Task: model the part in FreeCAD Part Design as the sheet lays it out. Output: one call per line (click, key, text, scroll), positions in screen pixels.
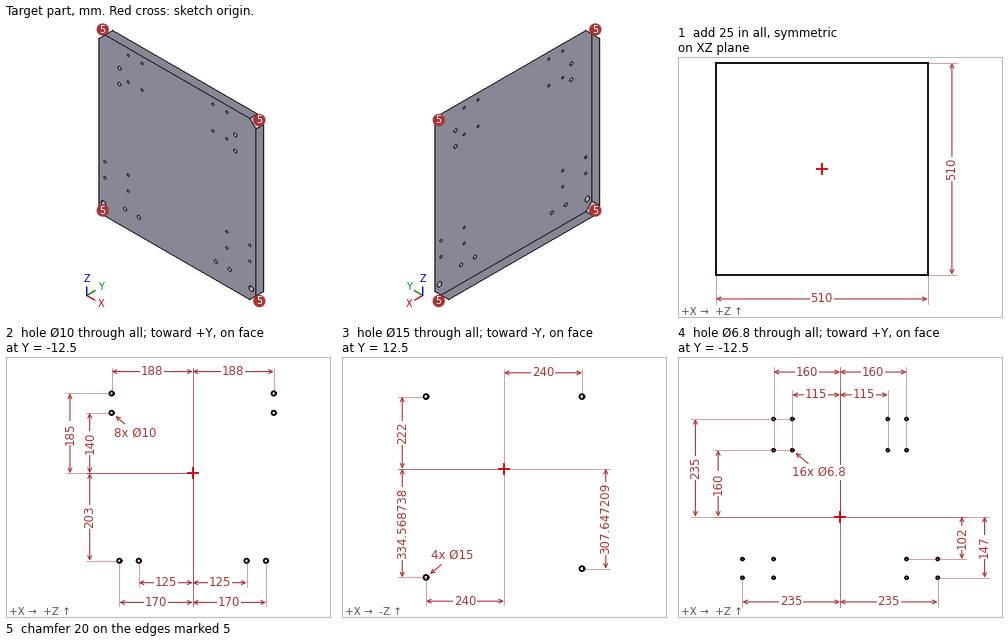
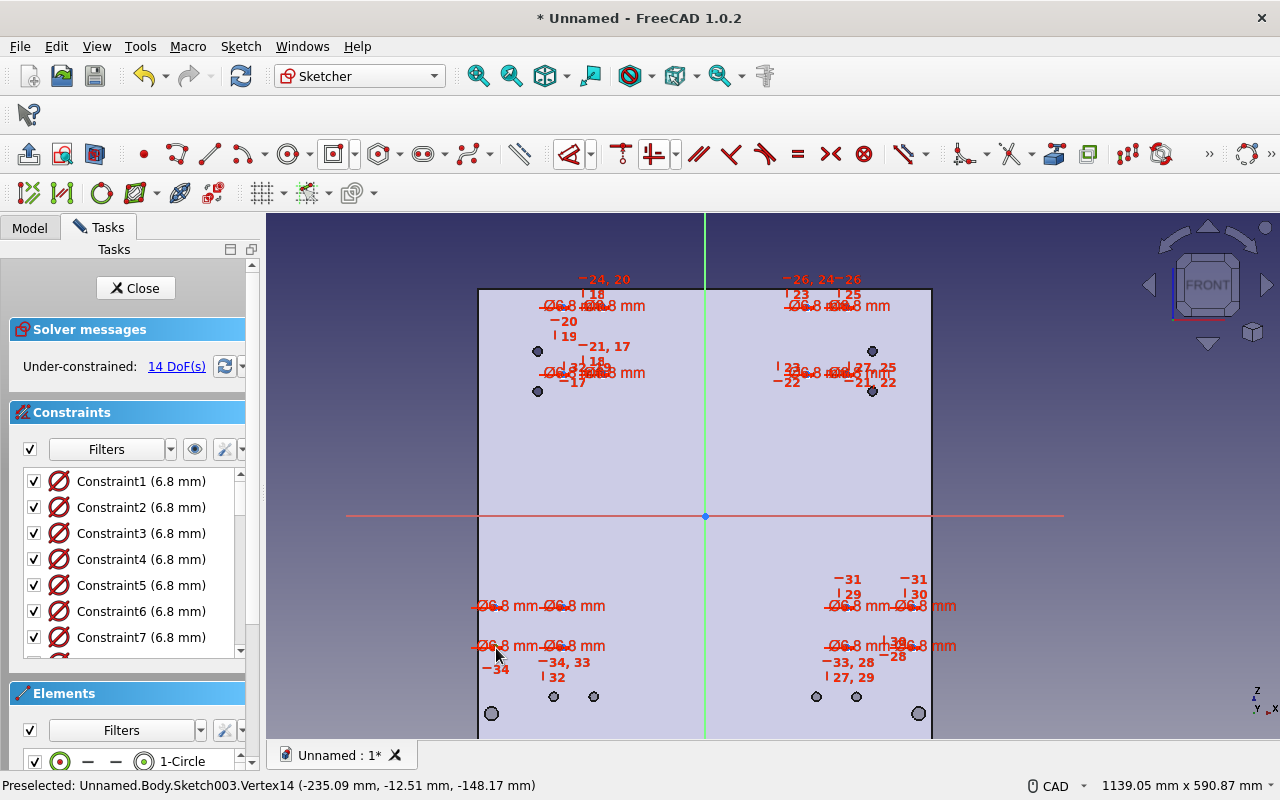
click(496, 608)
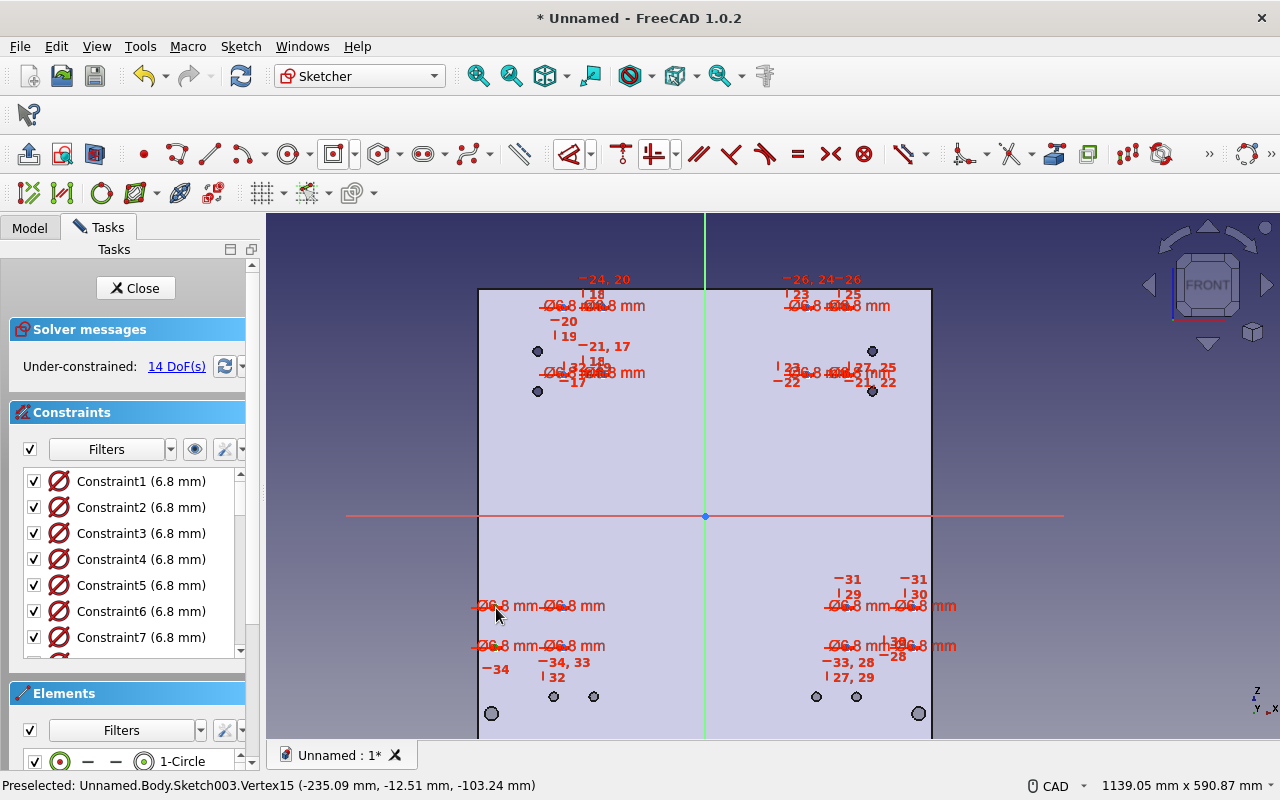
click(676, 154)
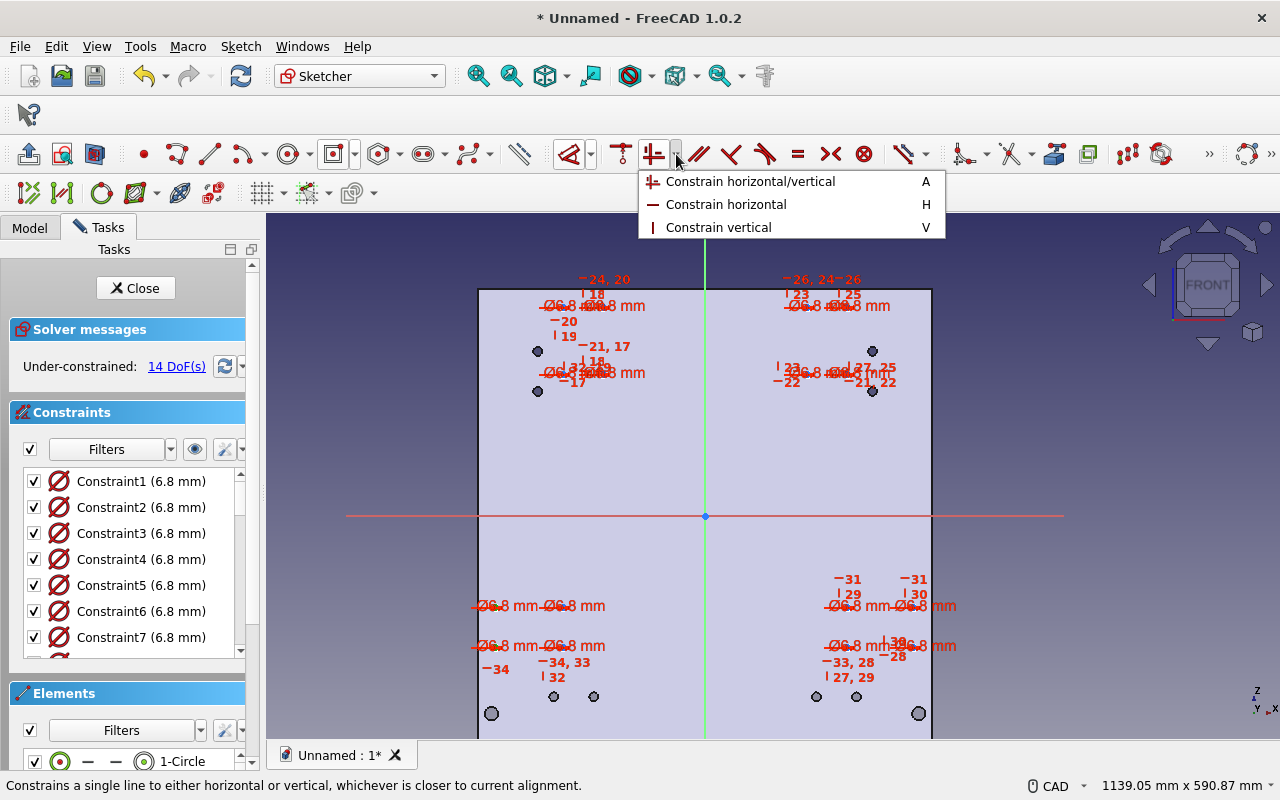
click(792, 228)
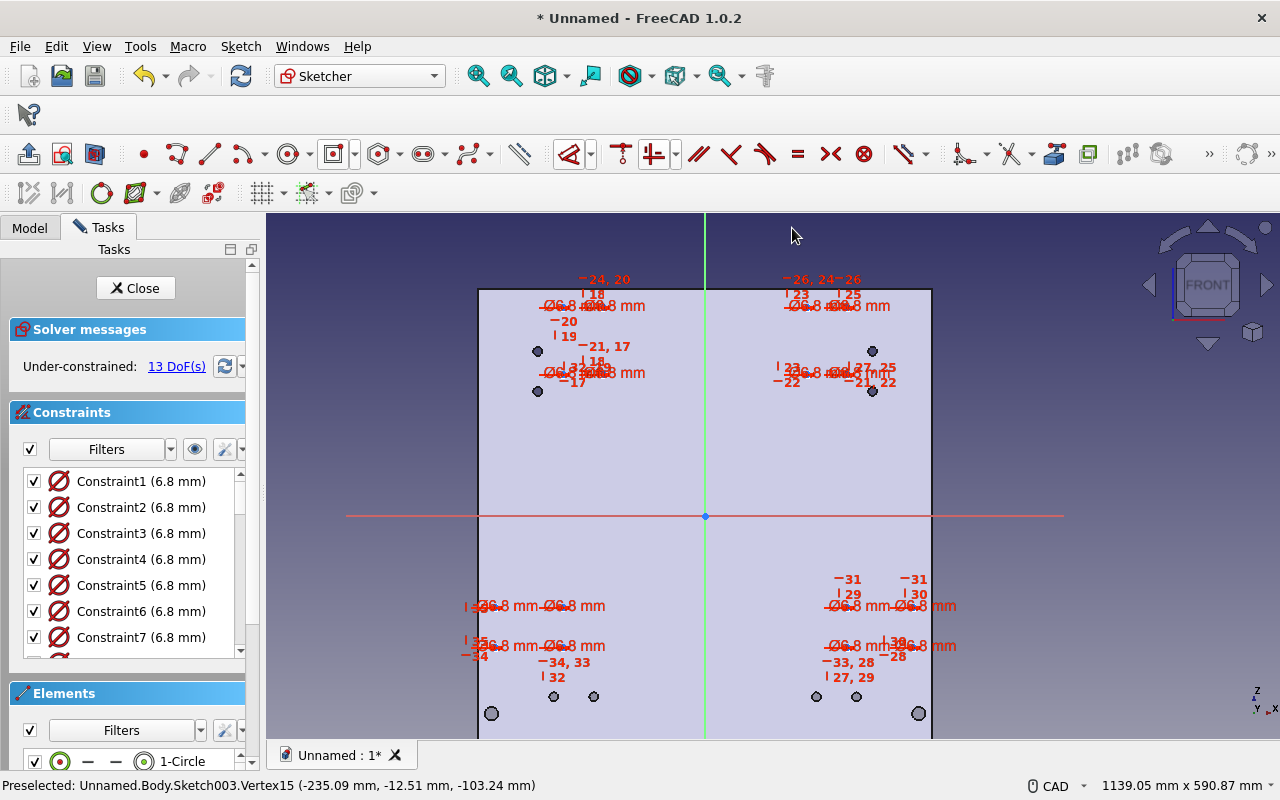
click(563, 648)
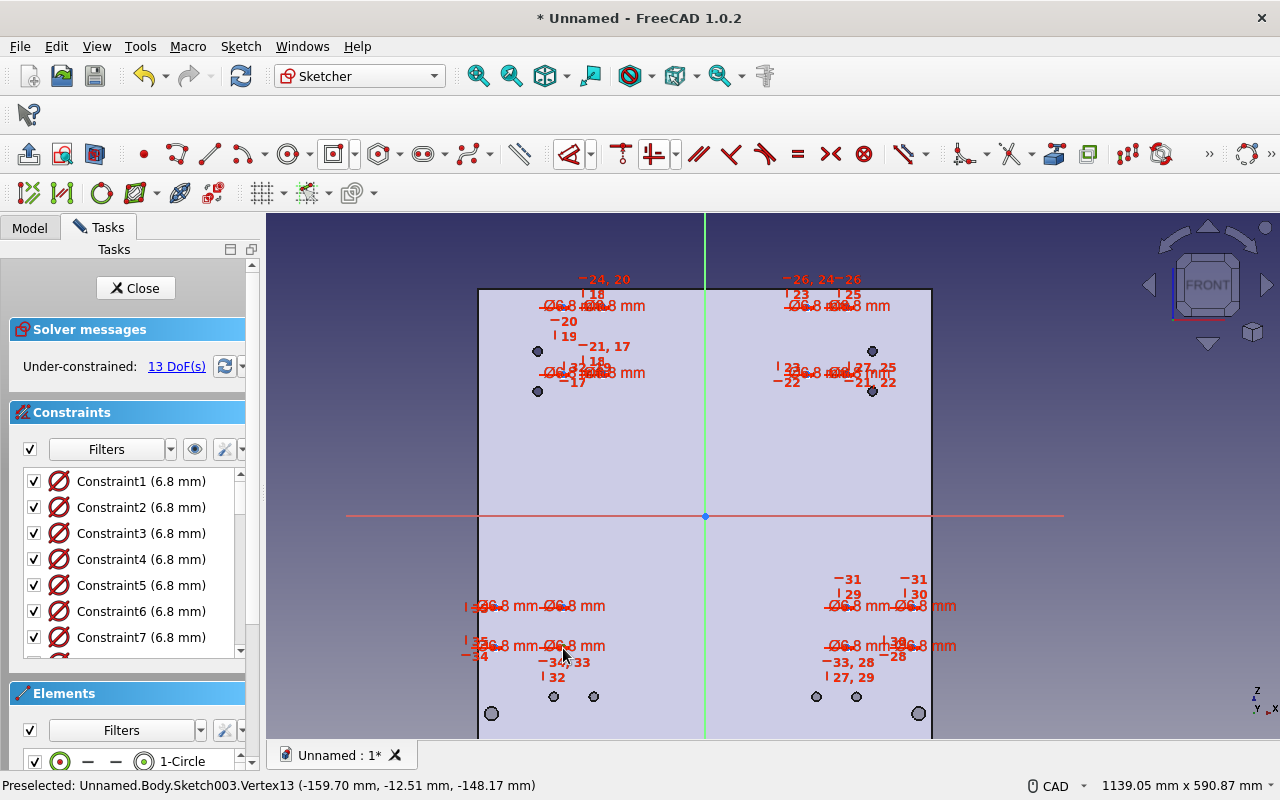
click(563, 608)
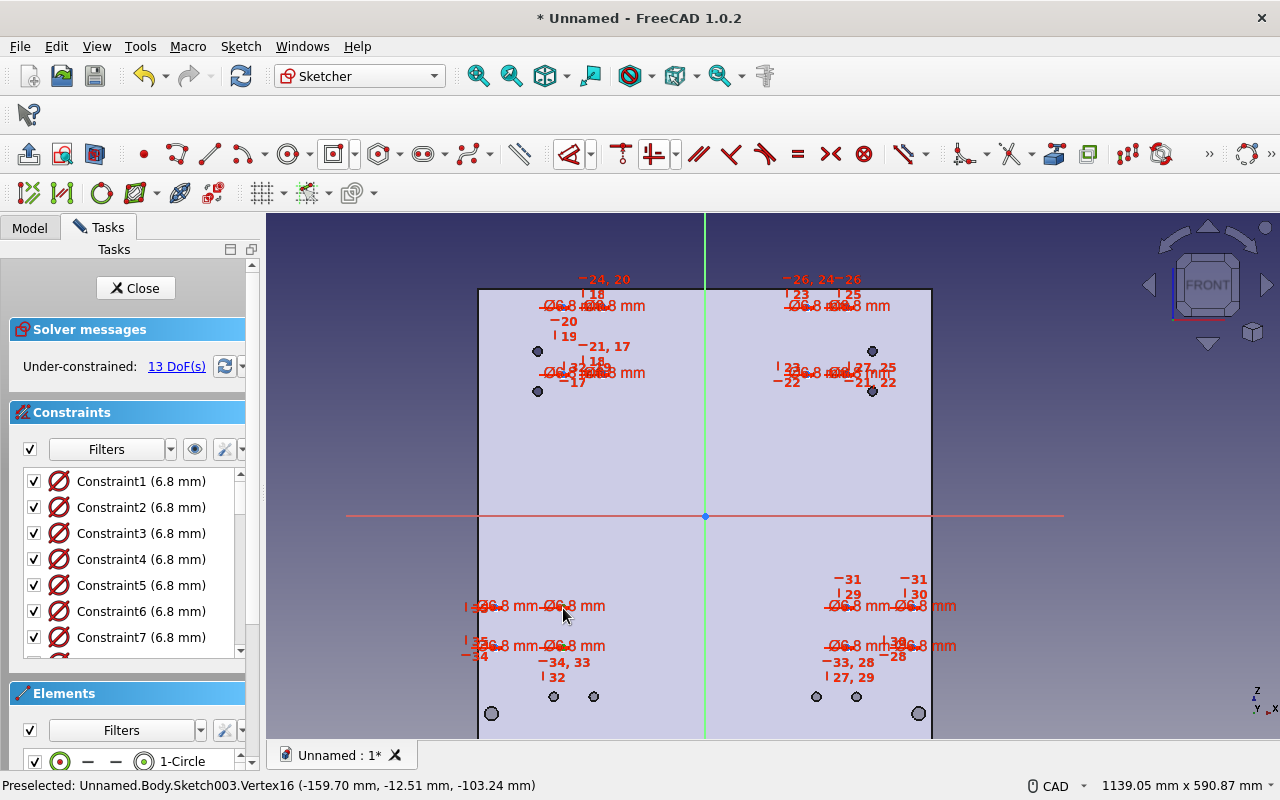
key(v)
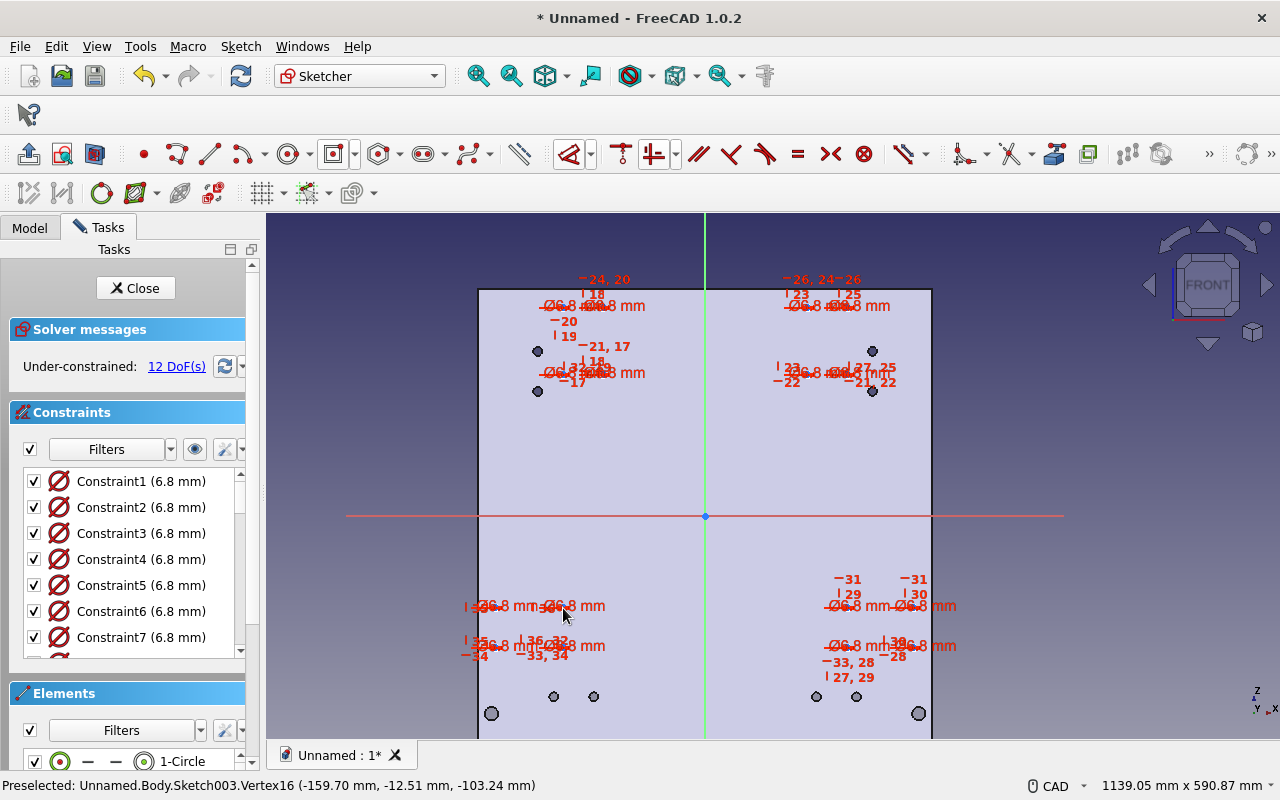
click(496, 608)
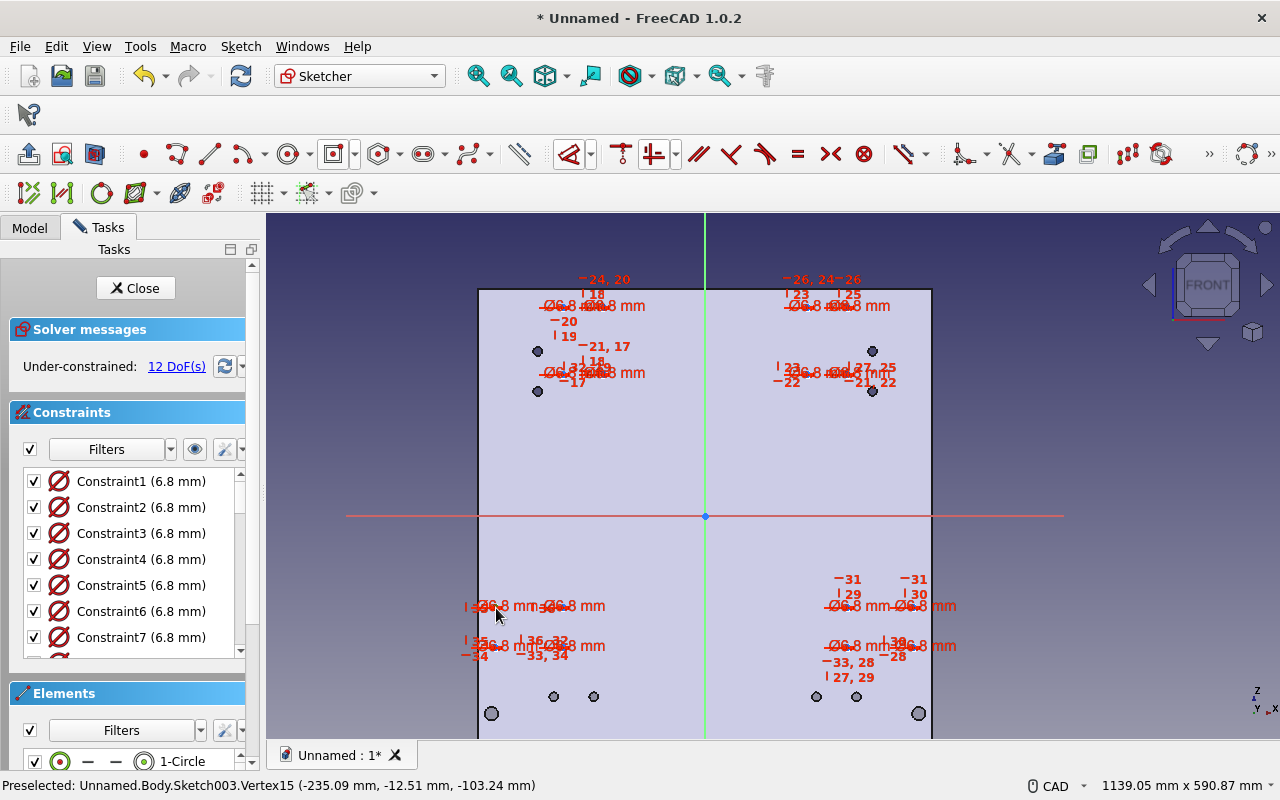
click(563, 608)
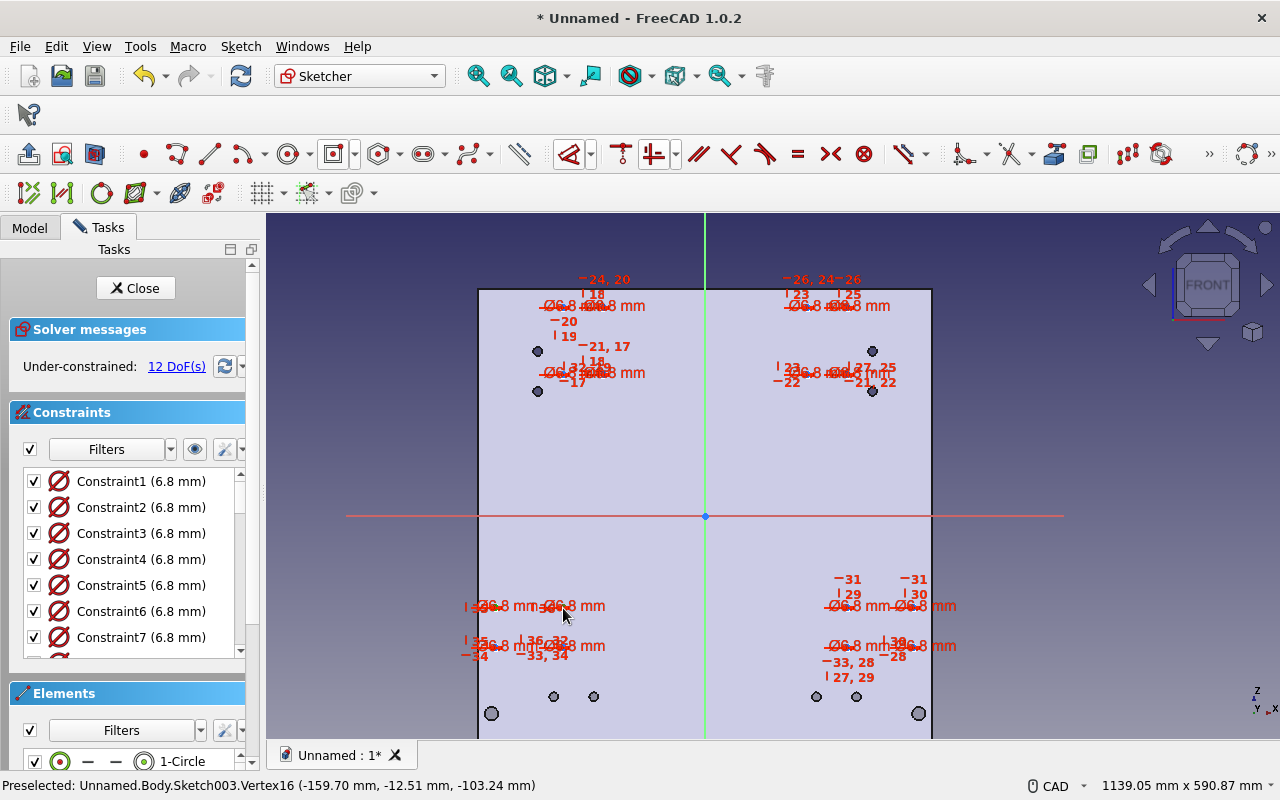
key(h)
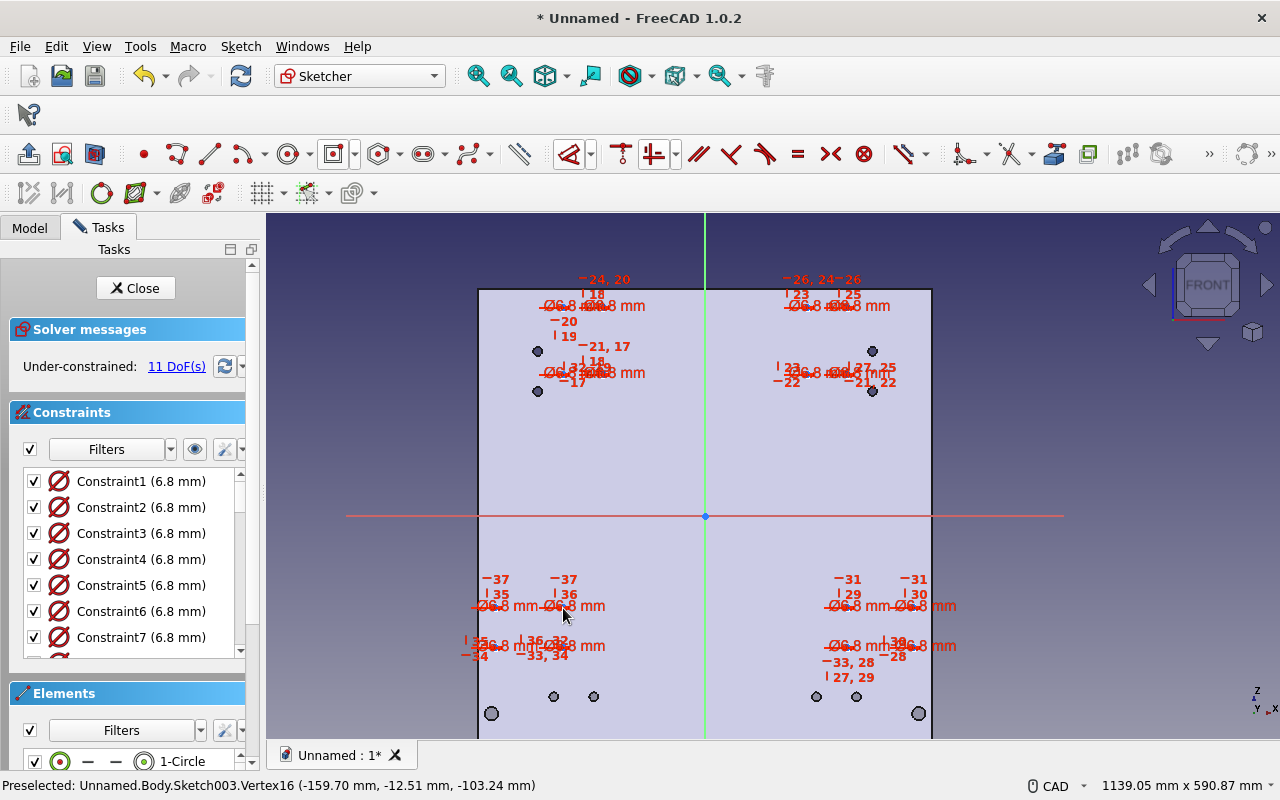
click(848, 608)